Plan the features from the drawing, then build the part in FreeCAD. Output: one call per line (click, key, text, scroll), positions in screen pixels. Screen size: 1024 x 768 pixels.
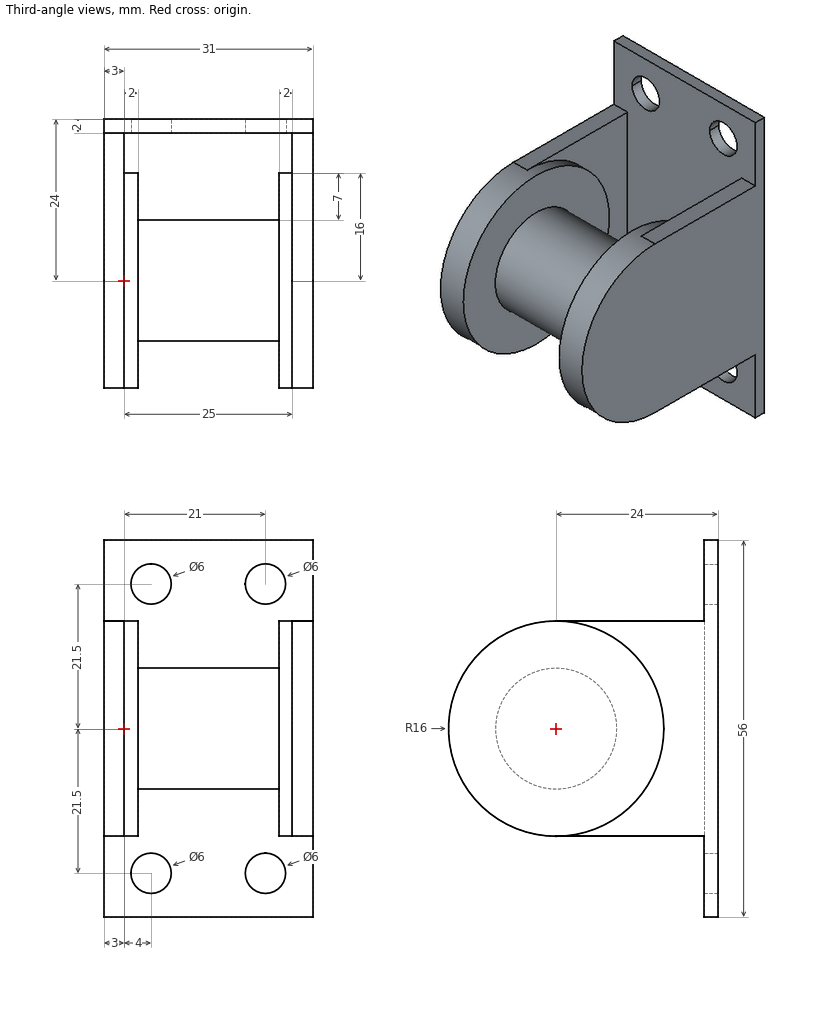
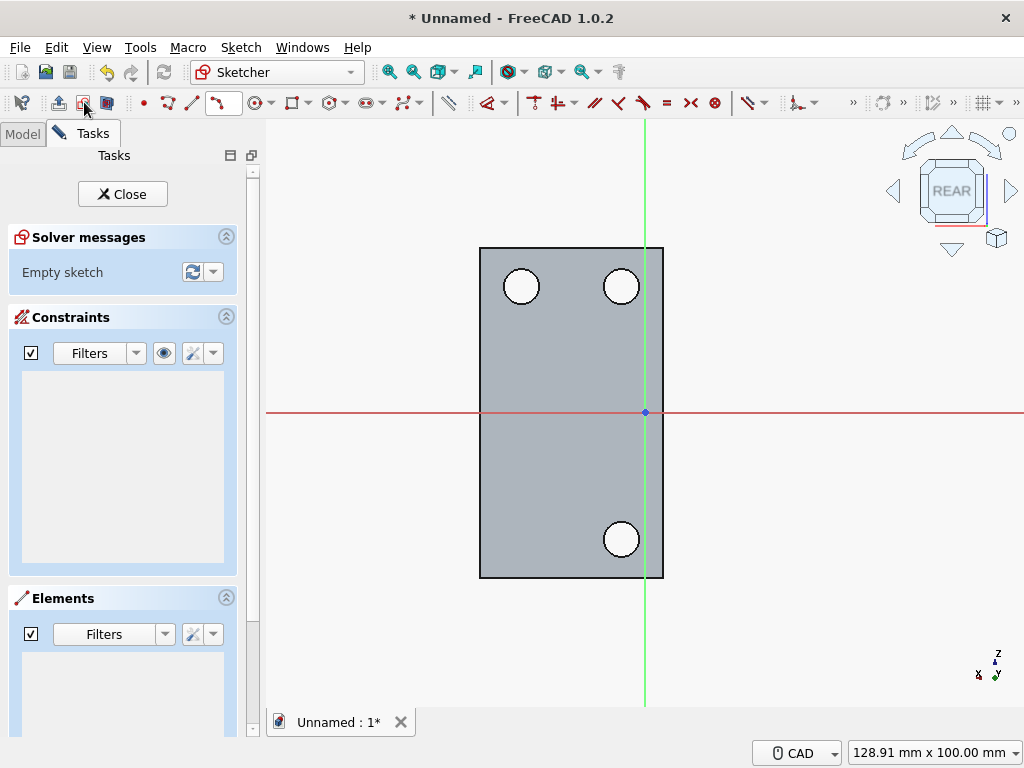
scroll(516, 552, up, 12)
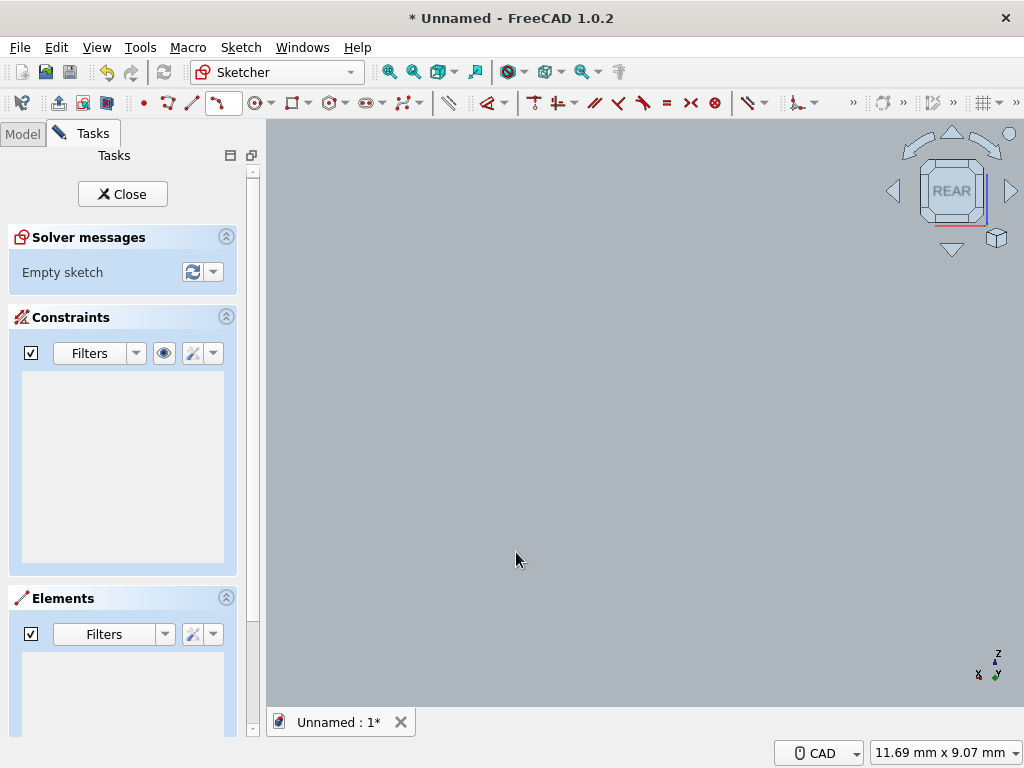
click(256, 104)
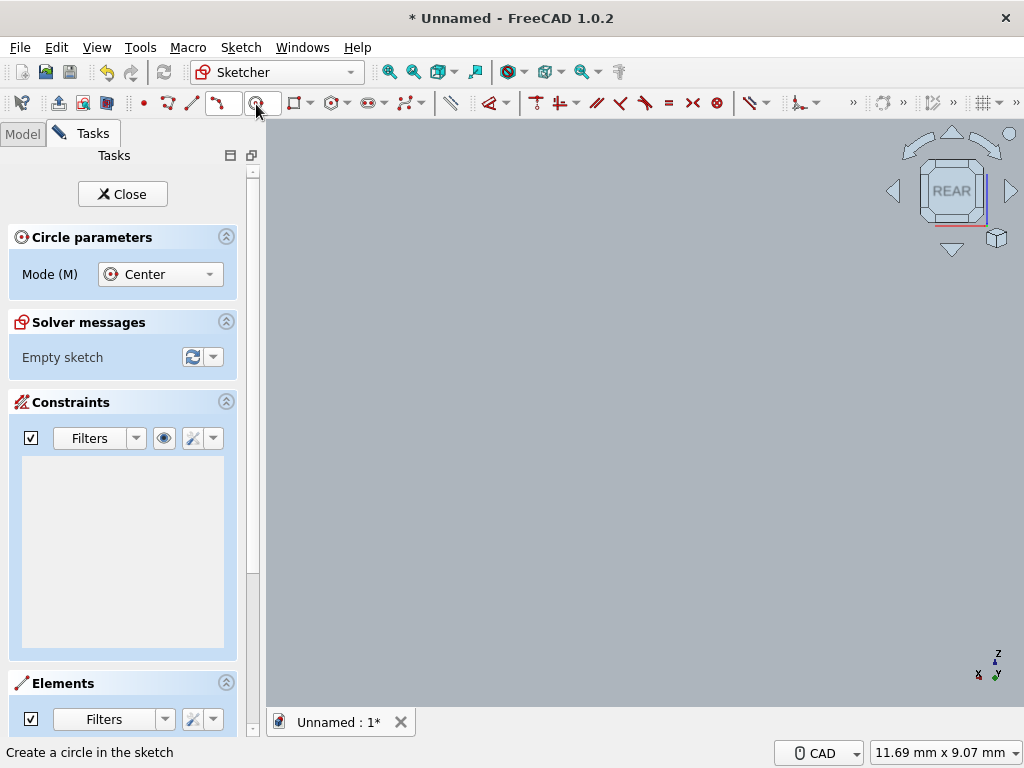
click(574, 406)
click(711, 268)
key(Escape)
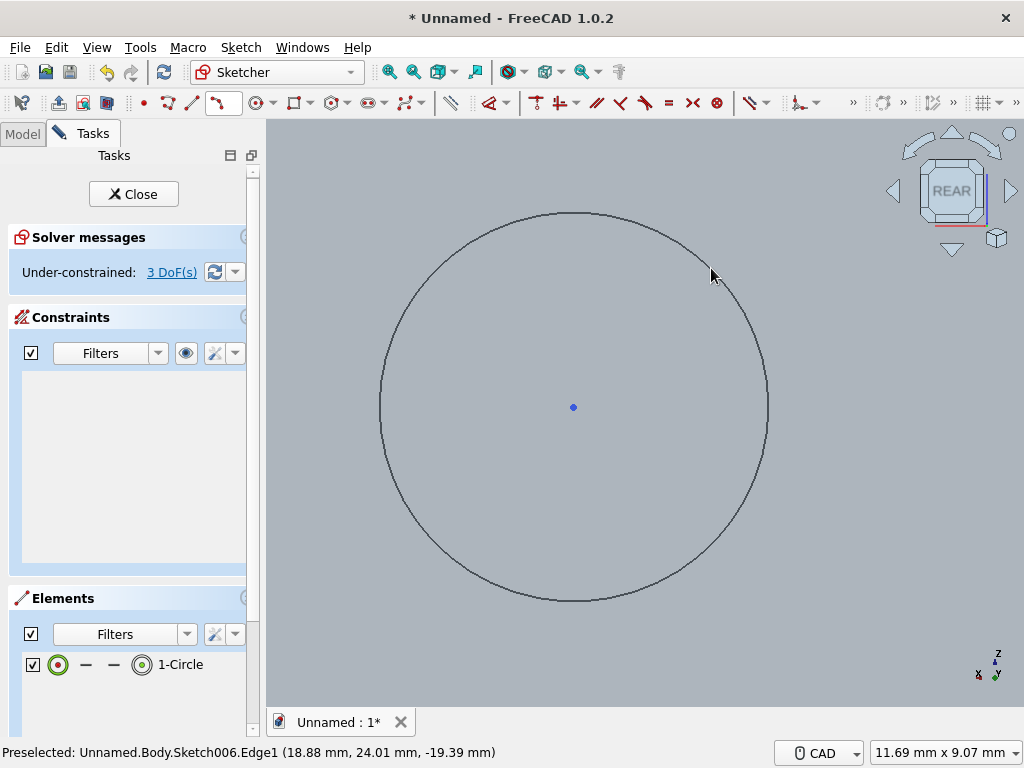
click(490, 104)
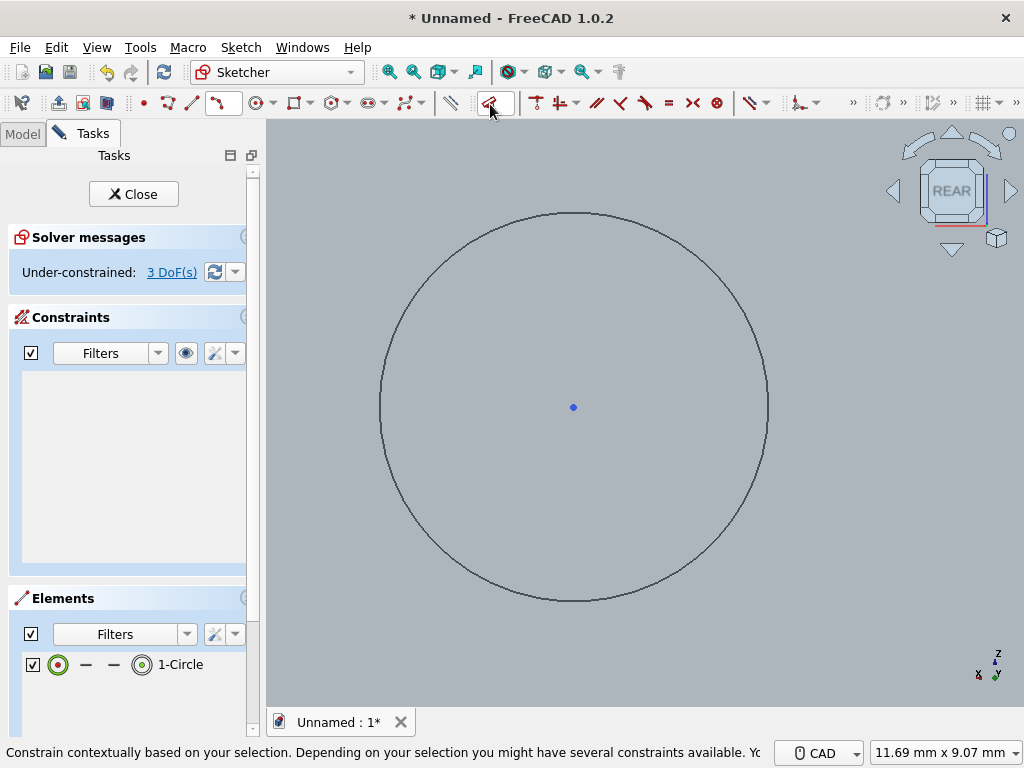
click(711, 269)
click(734, 246)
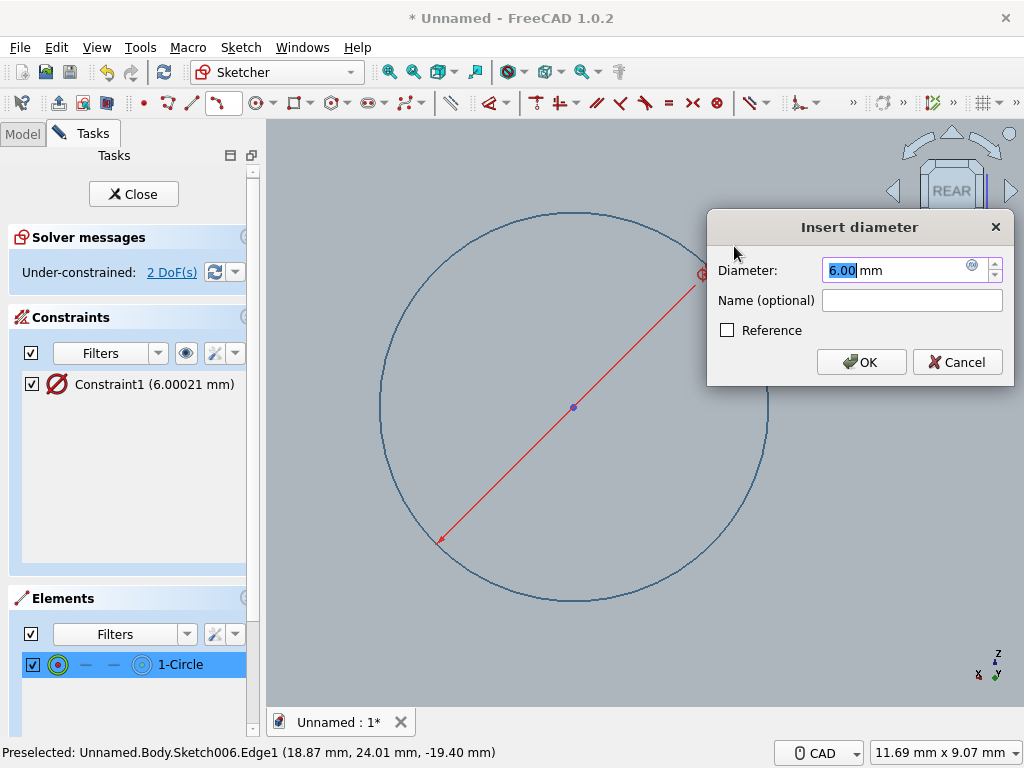
text(6)
key(Return)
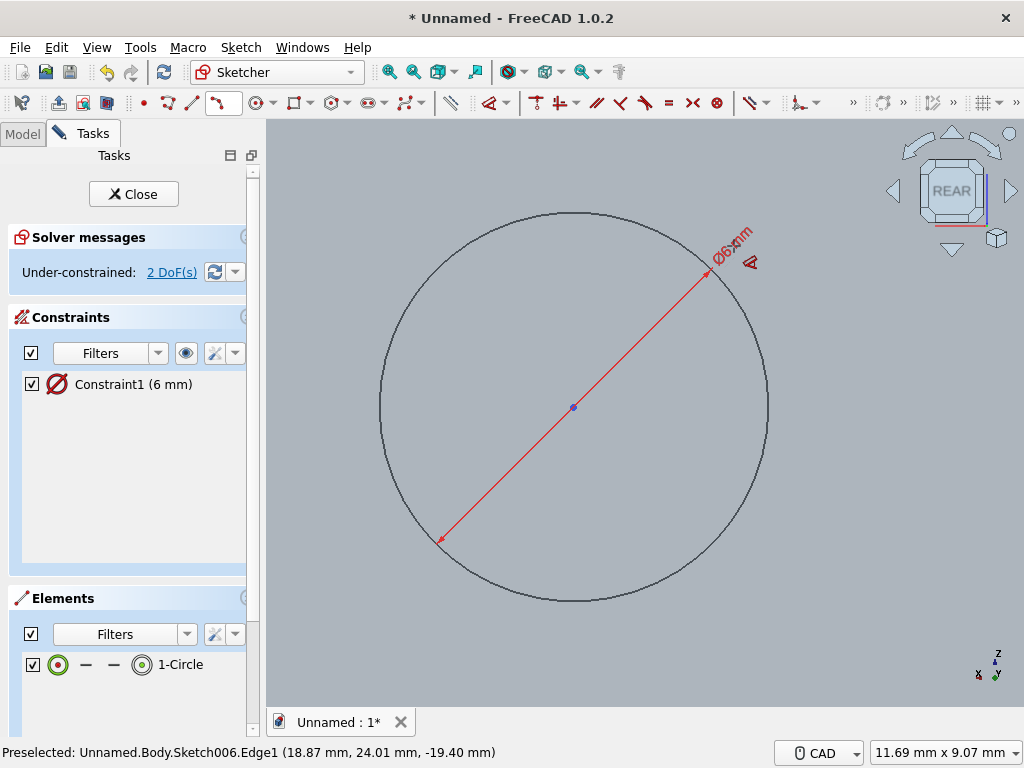
click(574, 407)
click(717, 441)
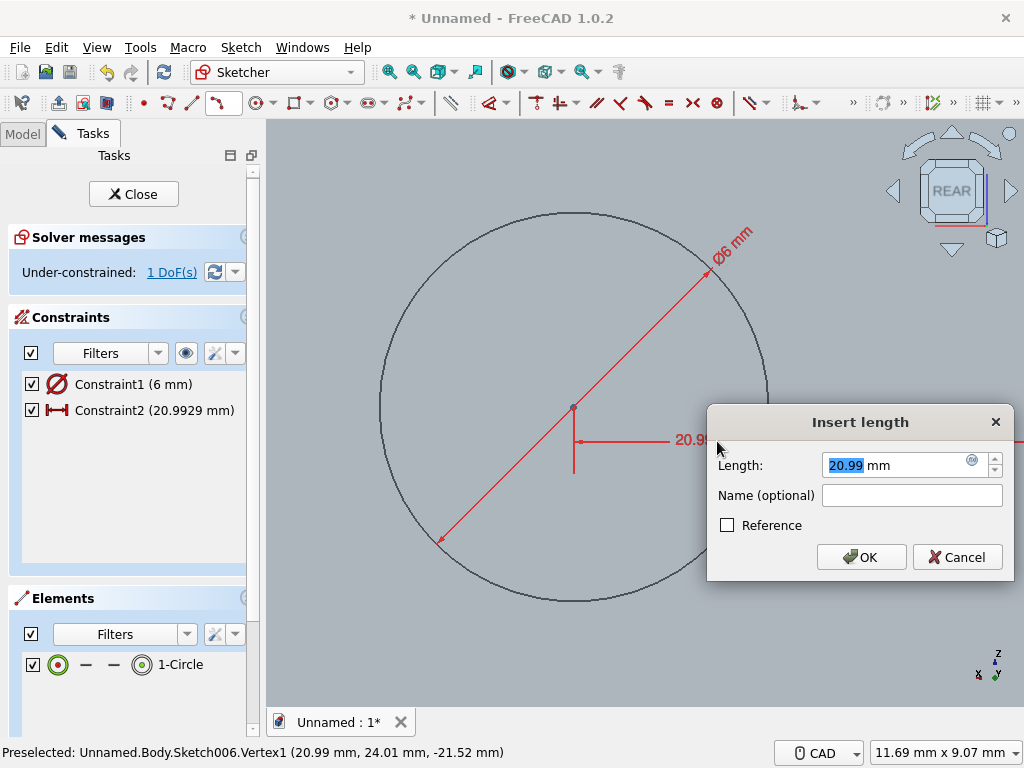
text(21)
key(Return)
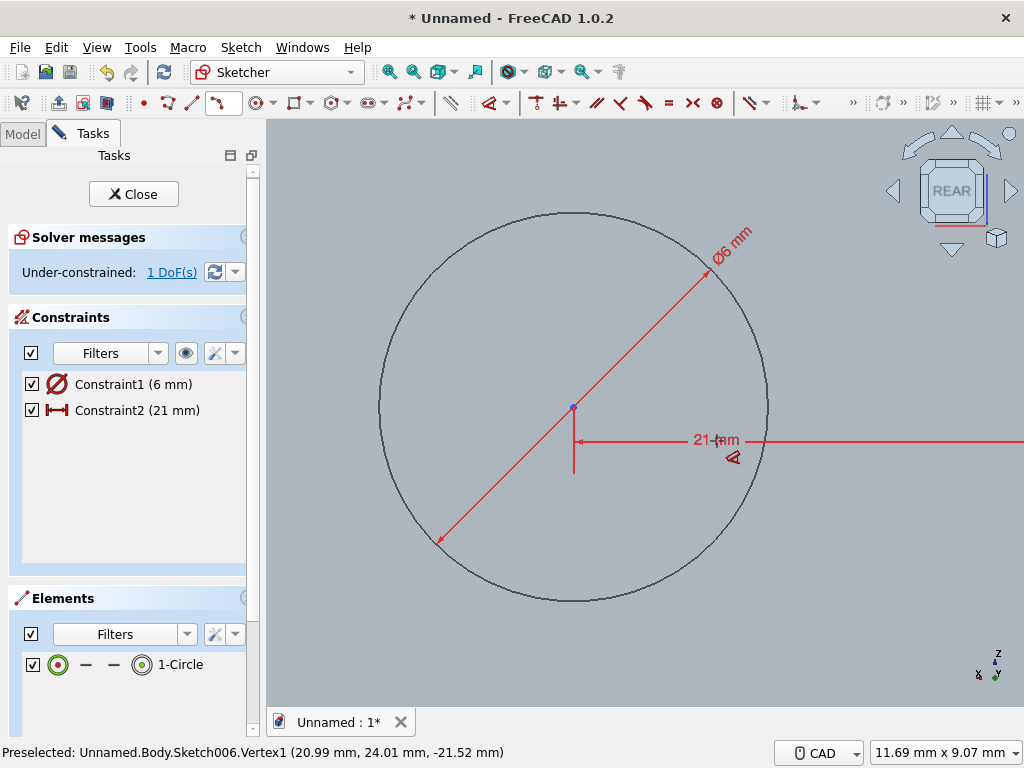
click(574, 407)
click(540, 277)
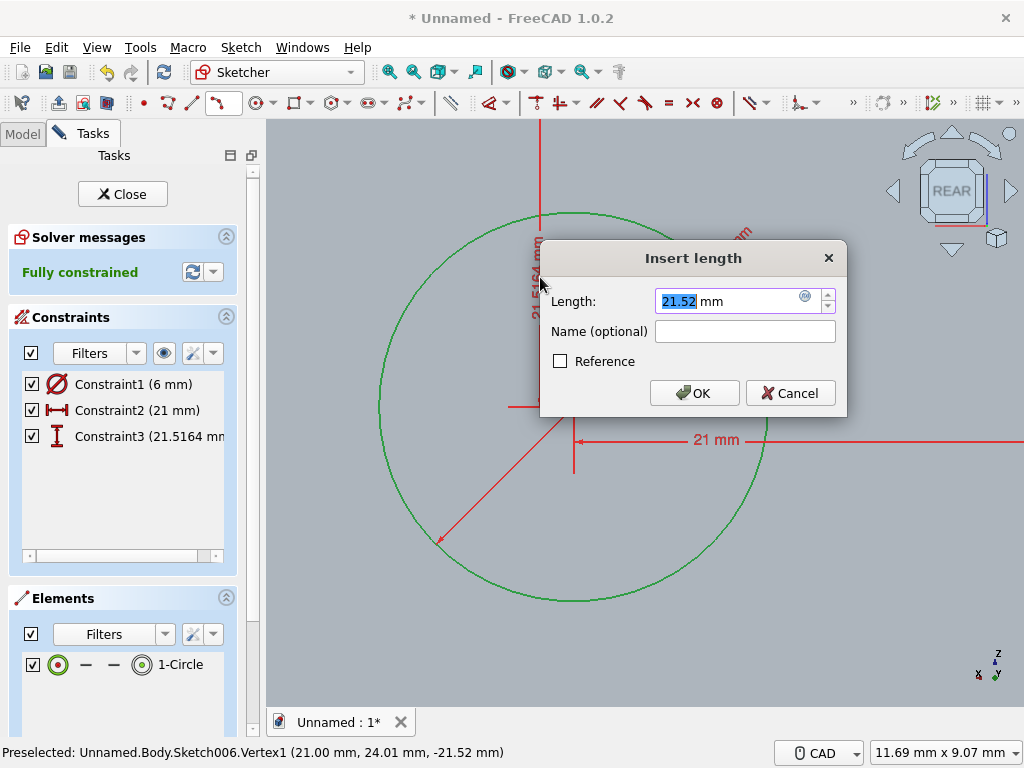
text(21.5)
key(Return)
key(Escape)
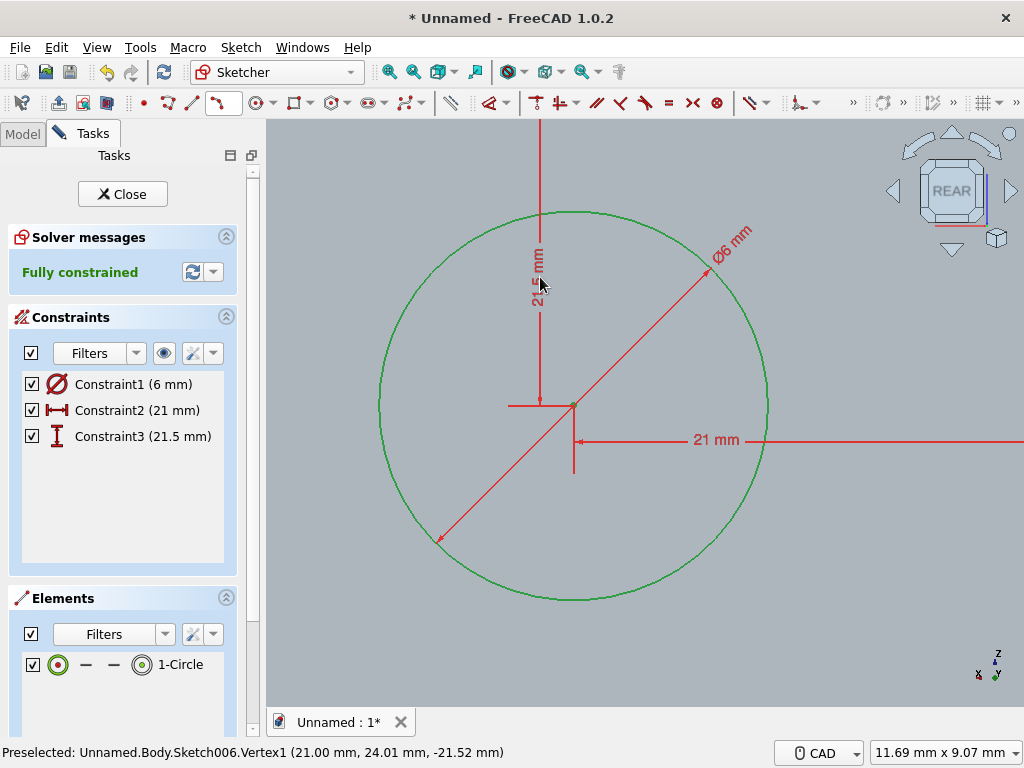
click(123, 194)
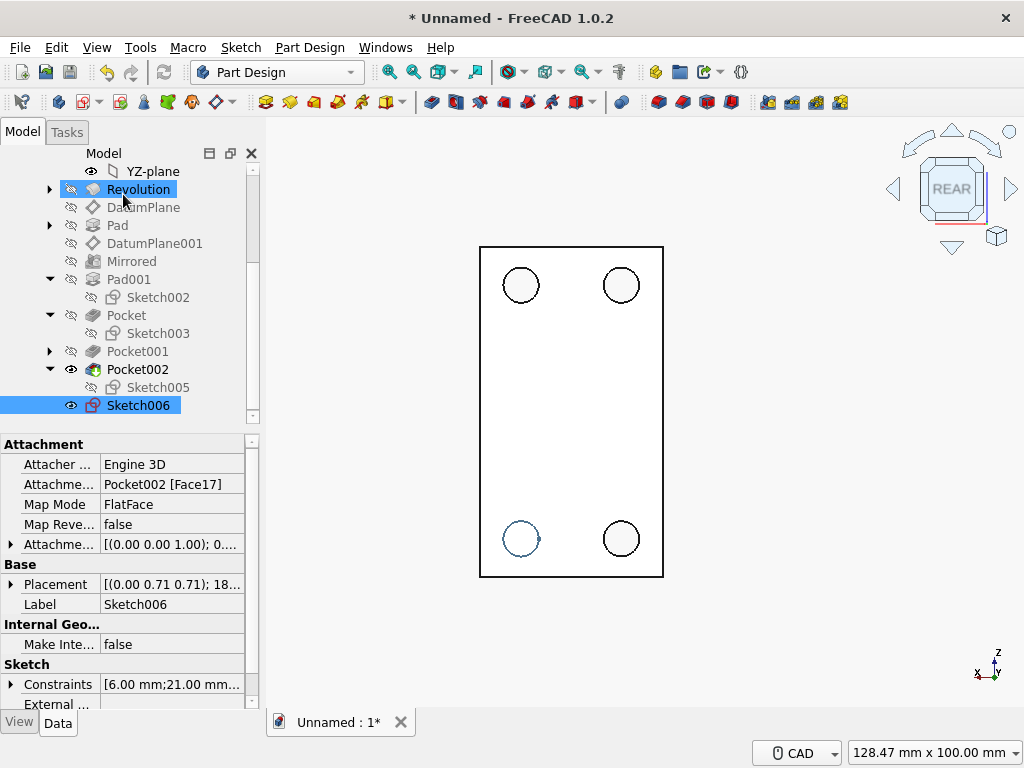
click(432, 102)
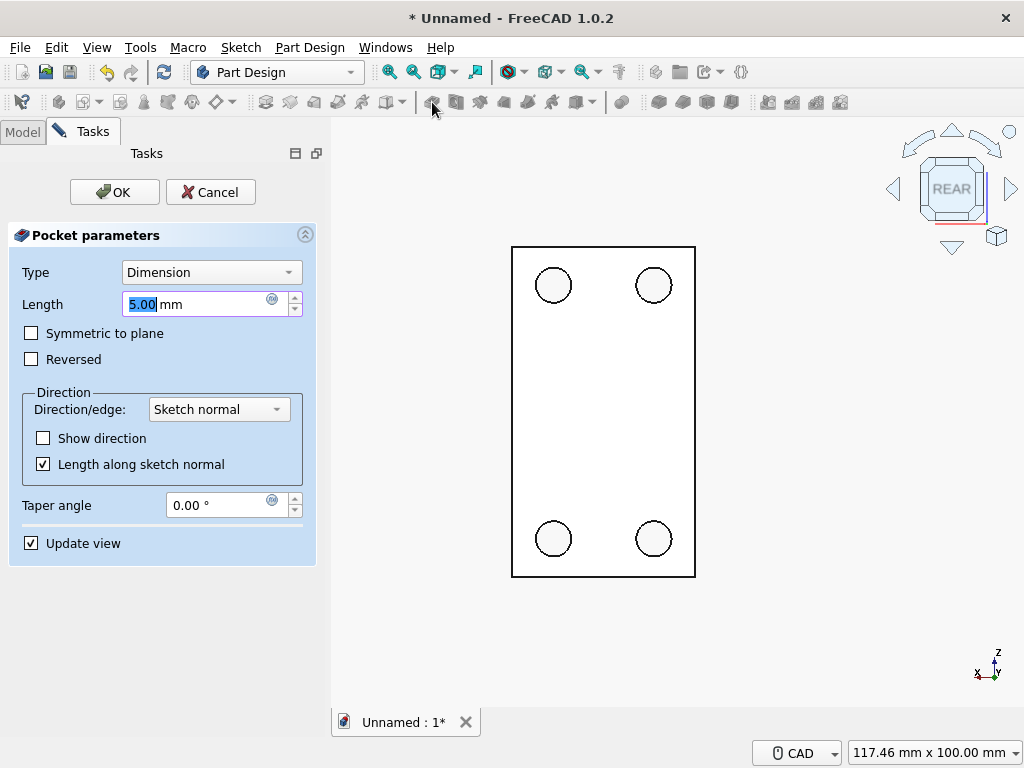
click(212, 272)